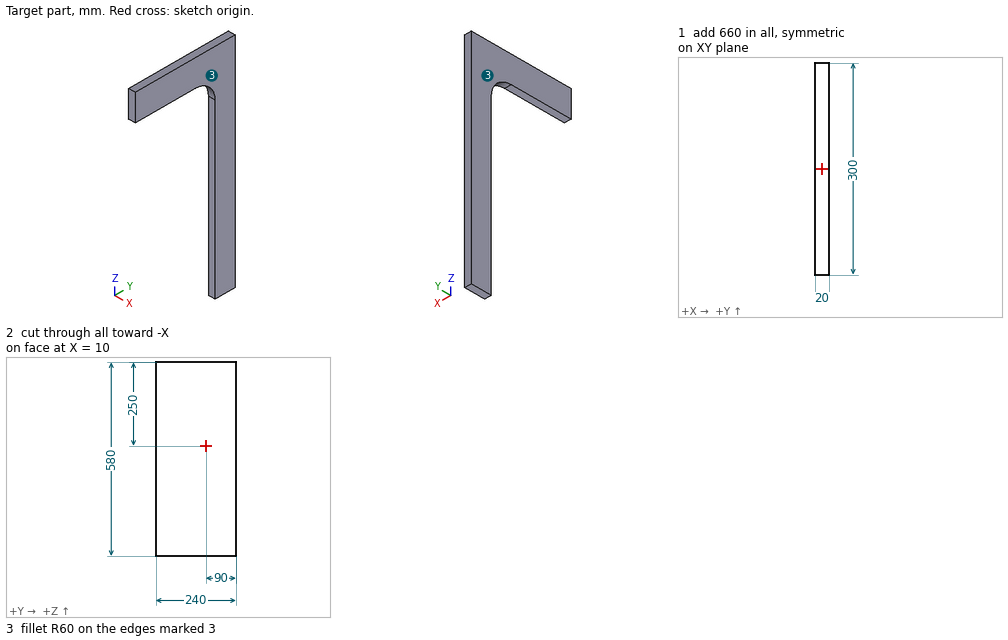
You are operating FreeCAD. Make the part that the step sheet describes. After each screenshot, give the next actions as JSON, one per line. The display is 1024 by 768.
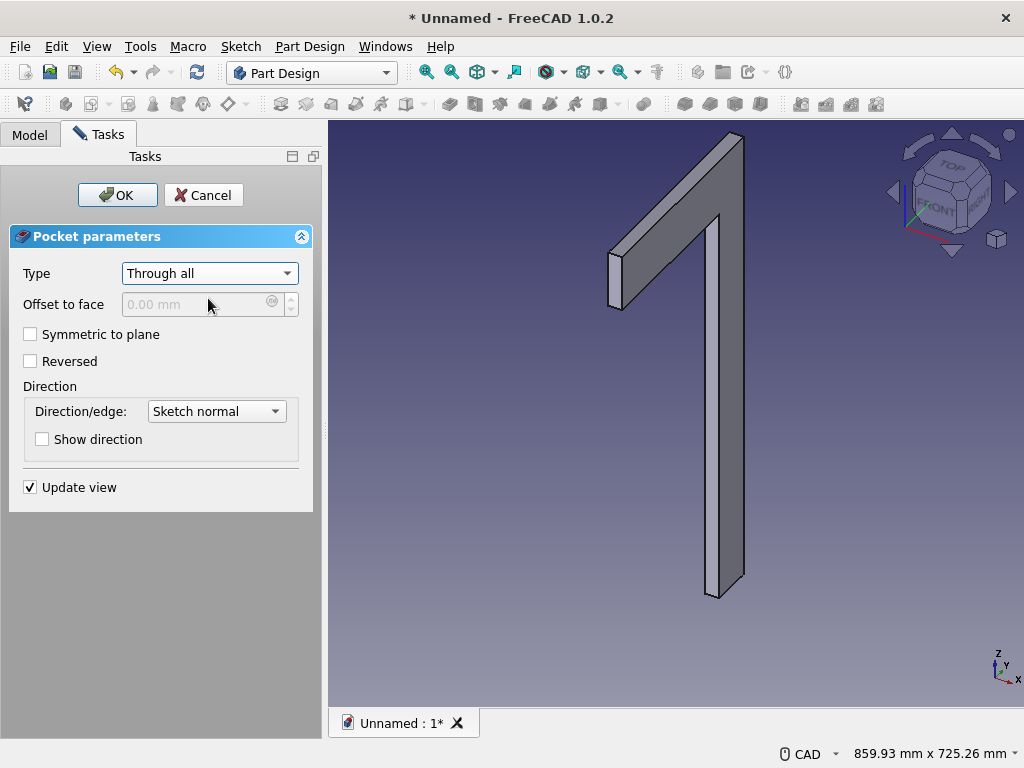
{"action": "left_click", "coordinate": [118, 195]}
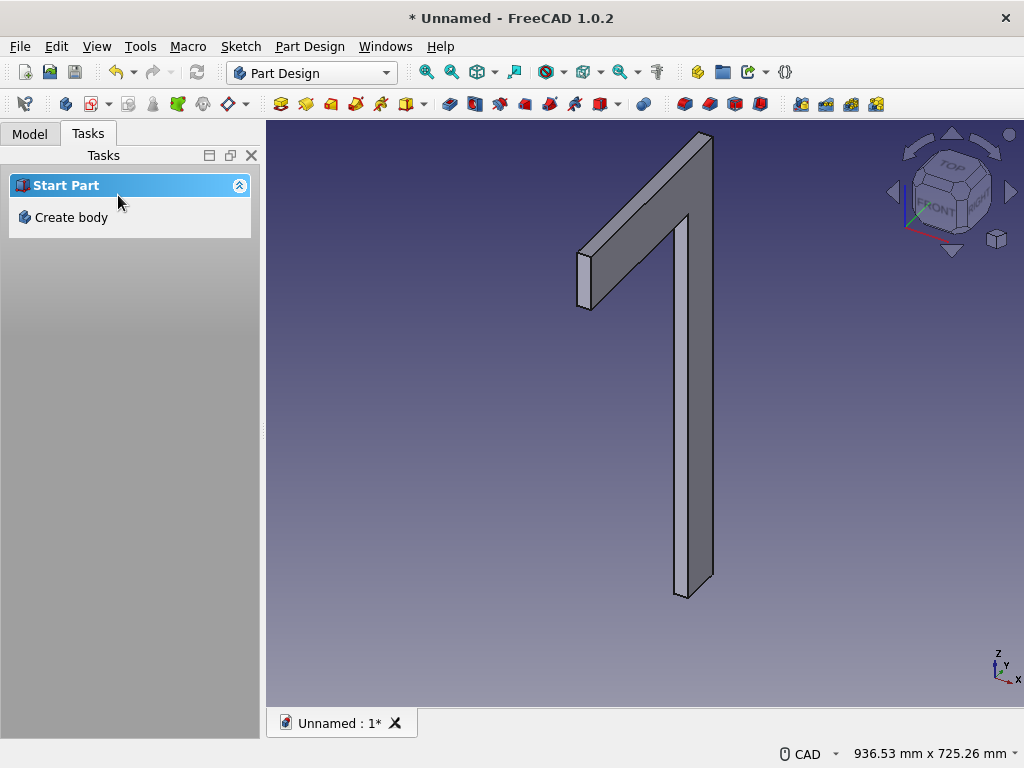
{"action": "scroll", "coordinate": [681, 211], "scroll_direction": "up", "scroll_amount": 5}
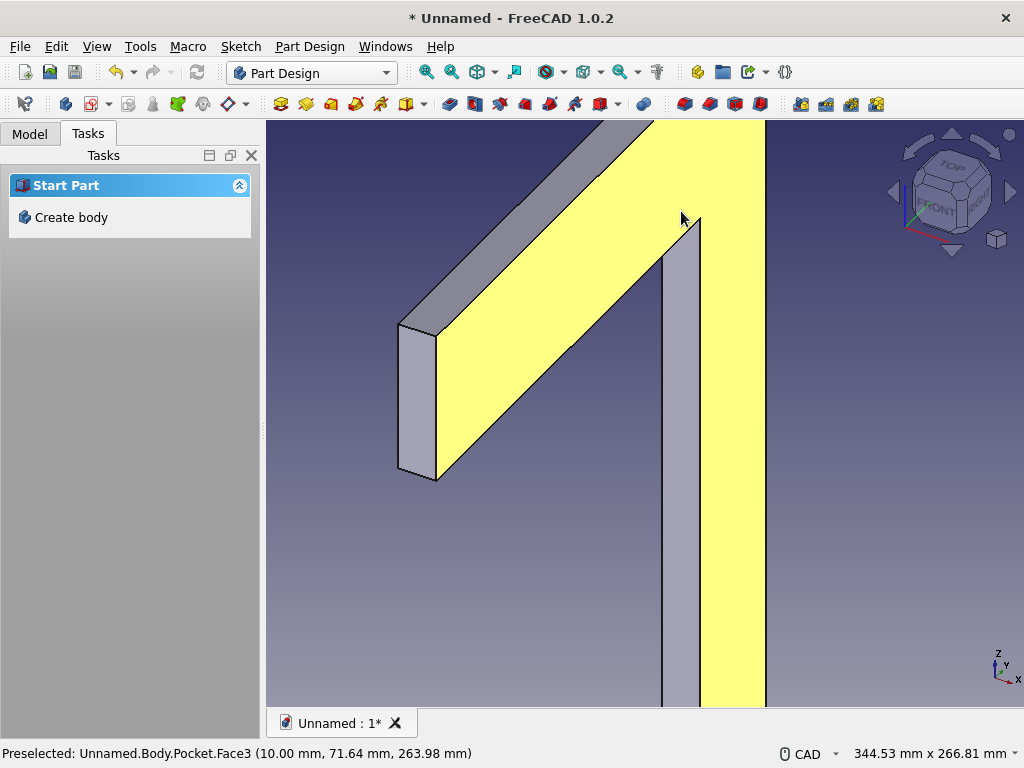
{"action": "left_click", "coordinate": [427, 72]}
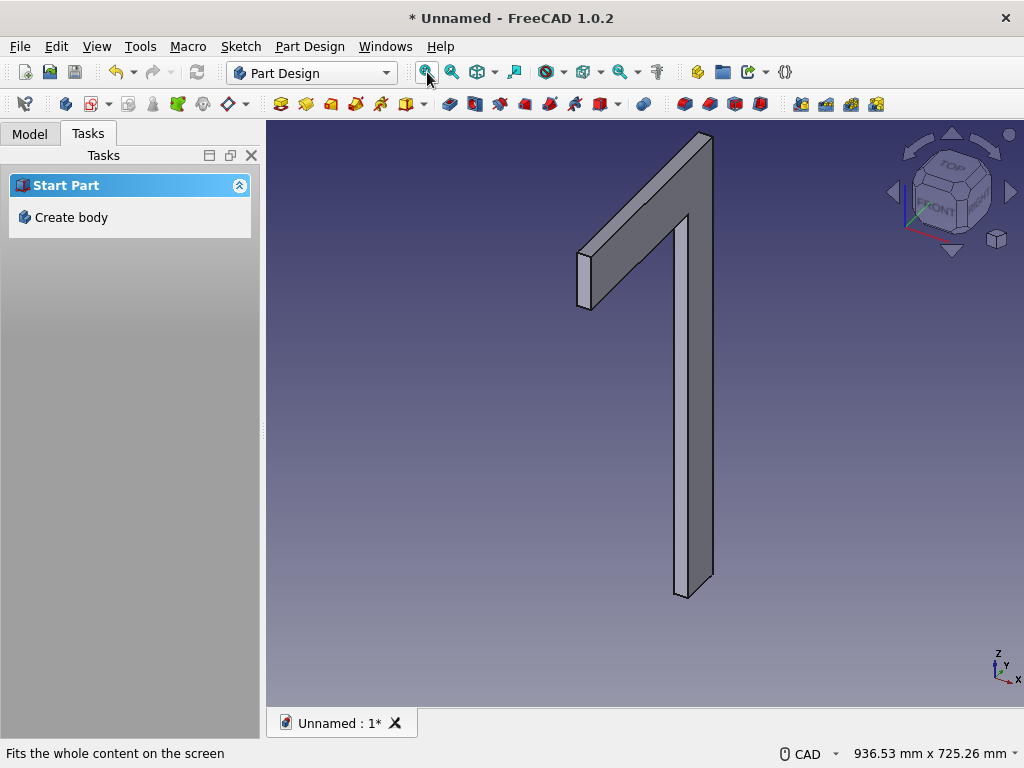
{"action": "key", "text": "0"}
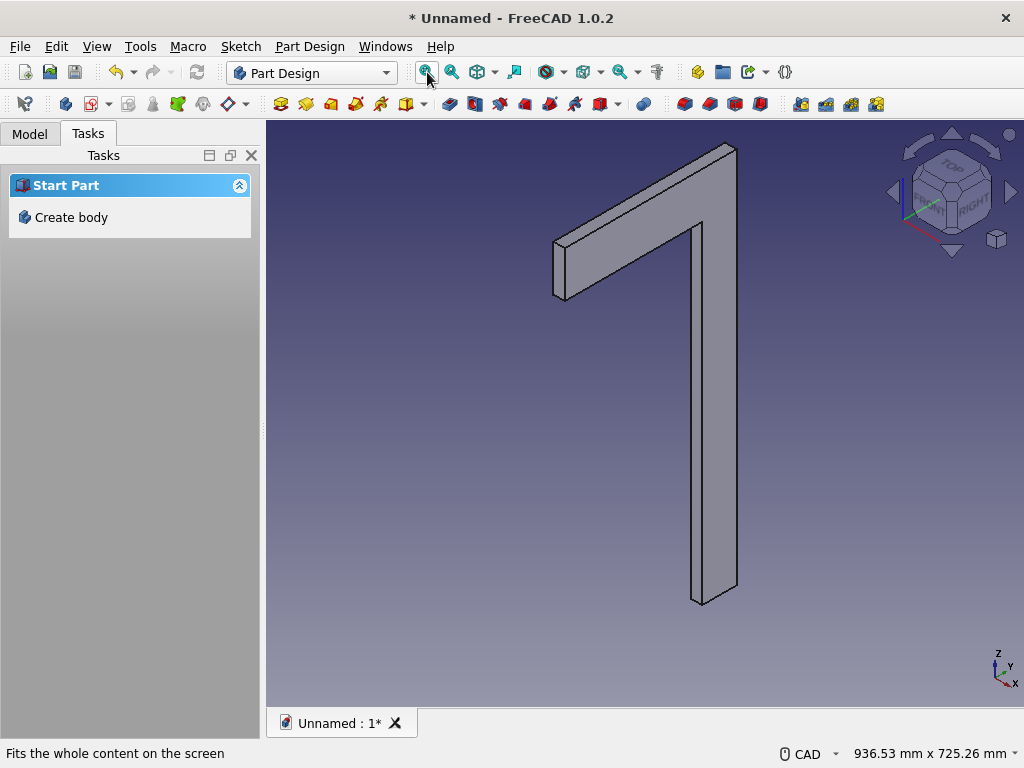
{"action": "scroll", "coordinate": [697, 218], "scroll_direction": "up", "scroll_amount": 5}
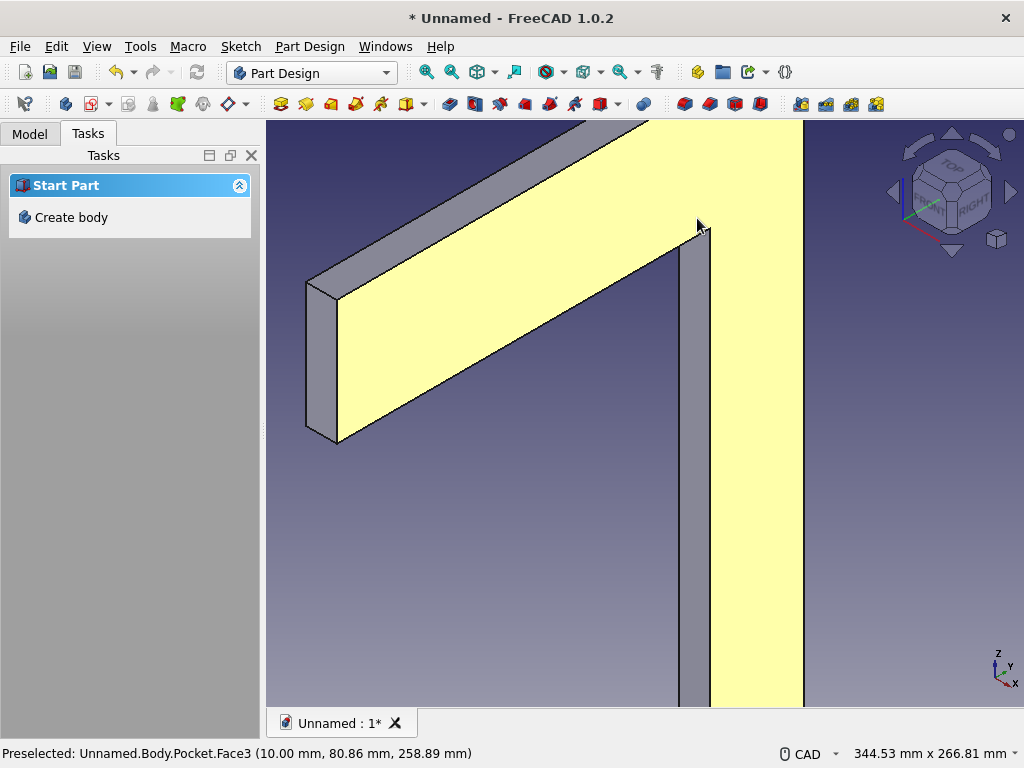
{"action": "left_click", "coordinate": [427, 72]}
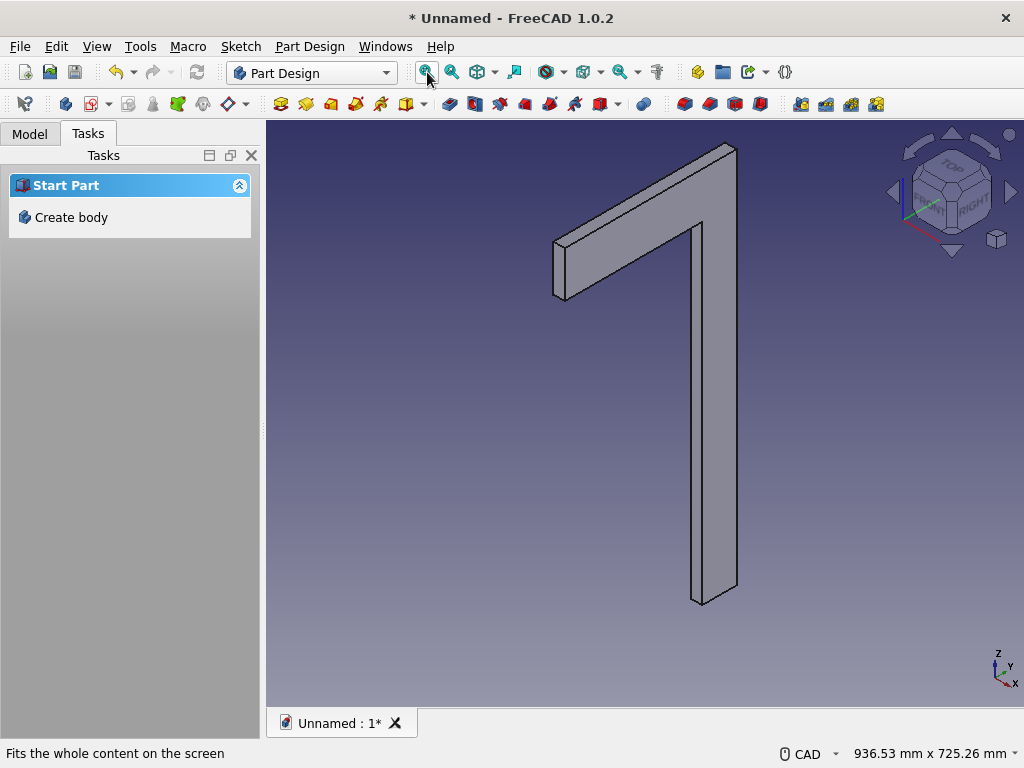
{"action": "key", "text": "2"}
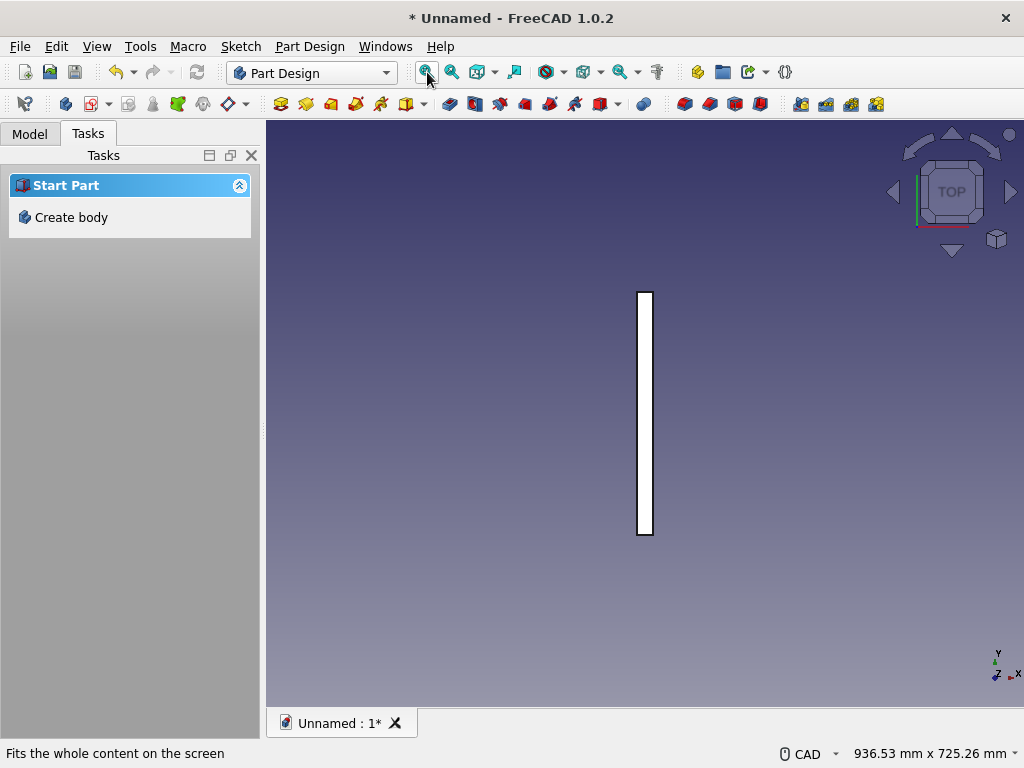
{"action": "left_click", "coordinate": [427, 72]}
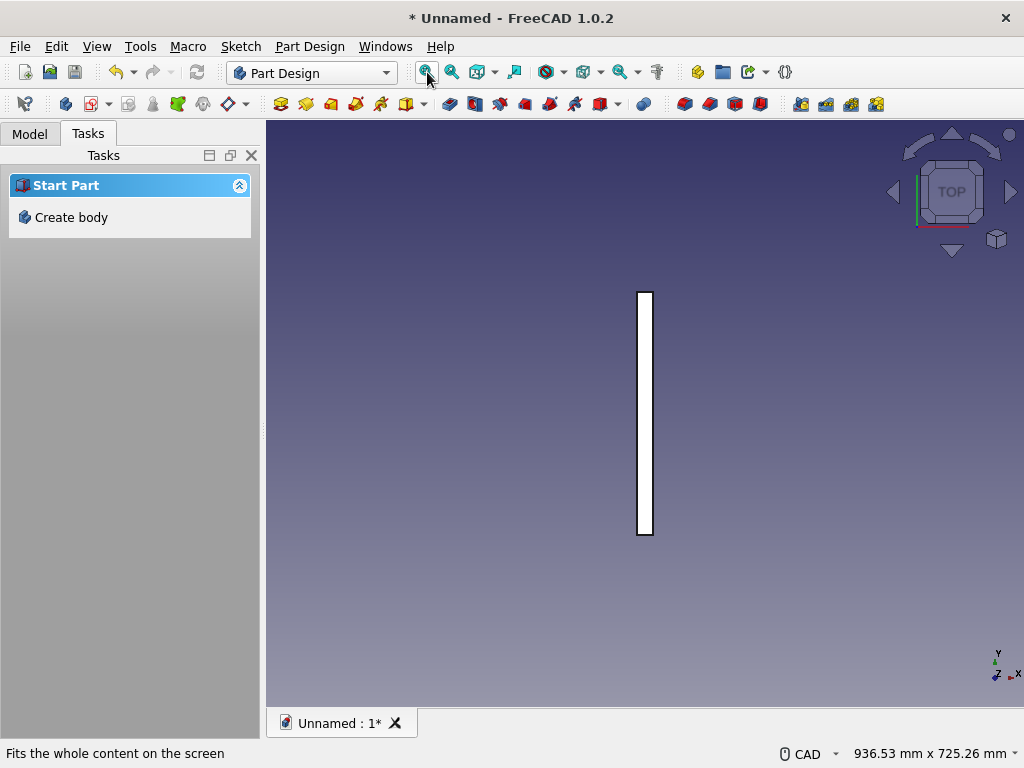
{"action": "scroll", "coordinate": [645, 340], "scroll_direction": "up", "scroll_amount": 5}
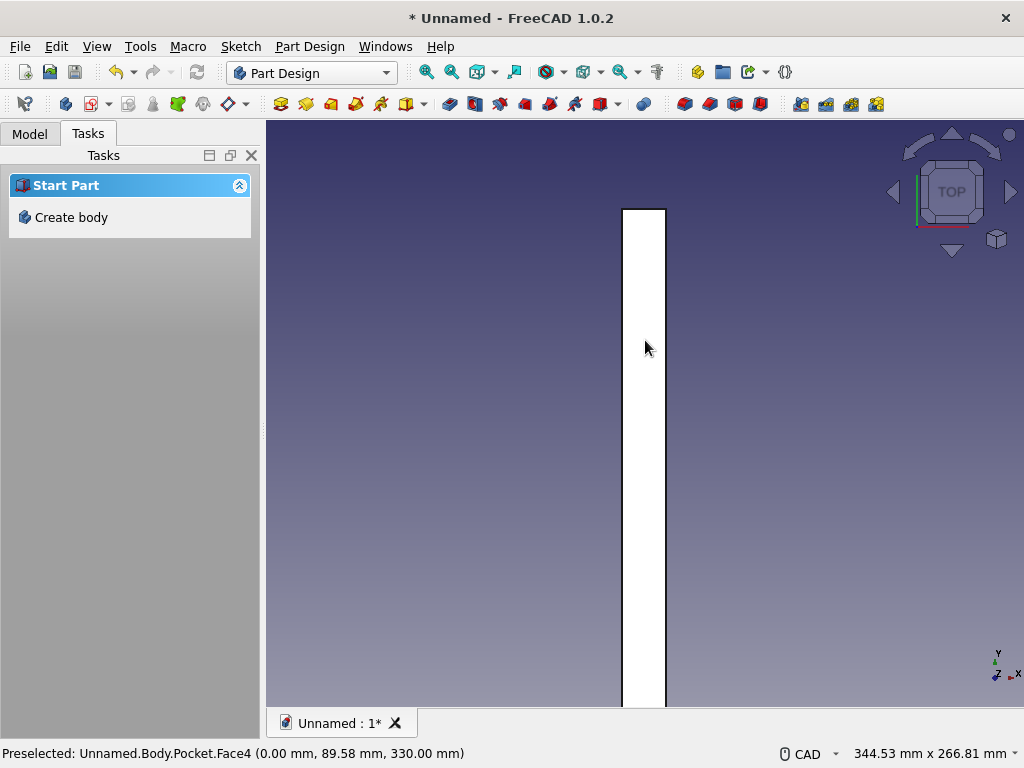
{"action": "key", "text": "v f"}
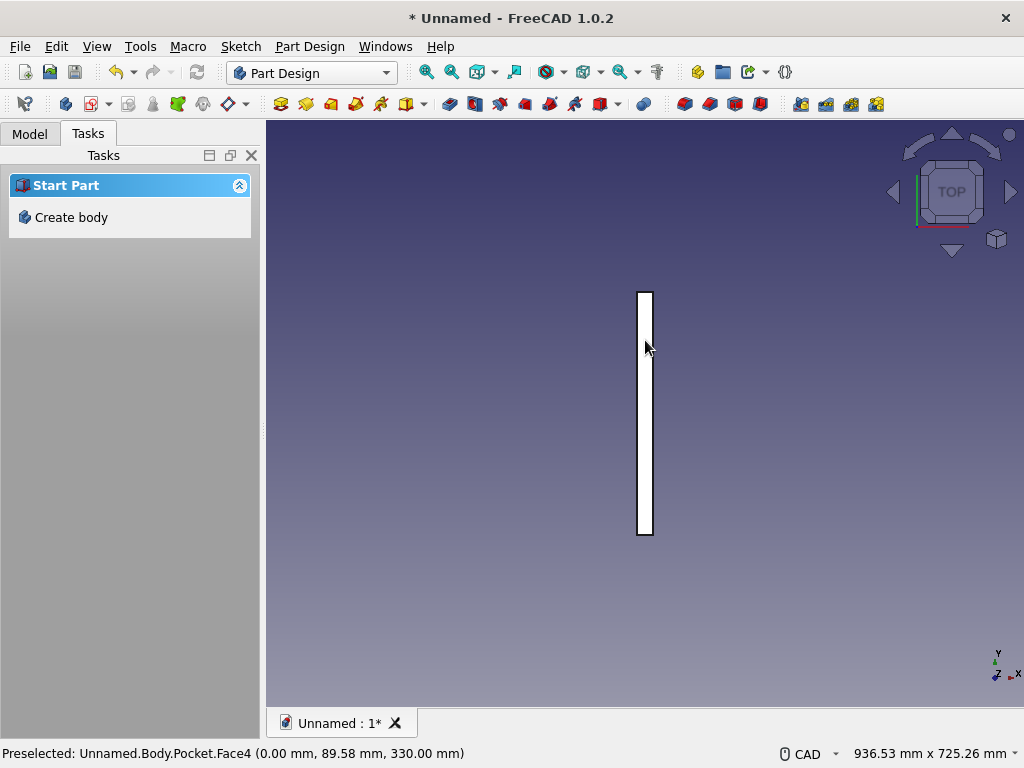
{"action": "key", "text": "1"}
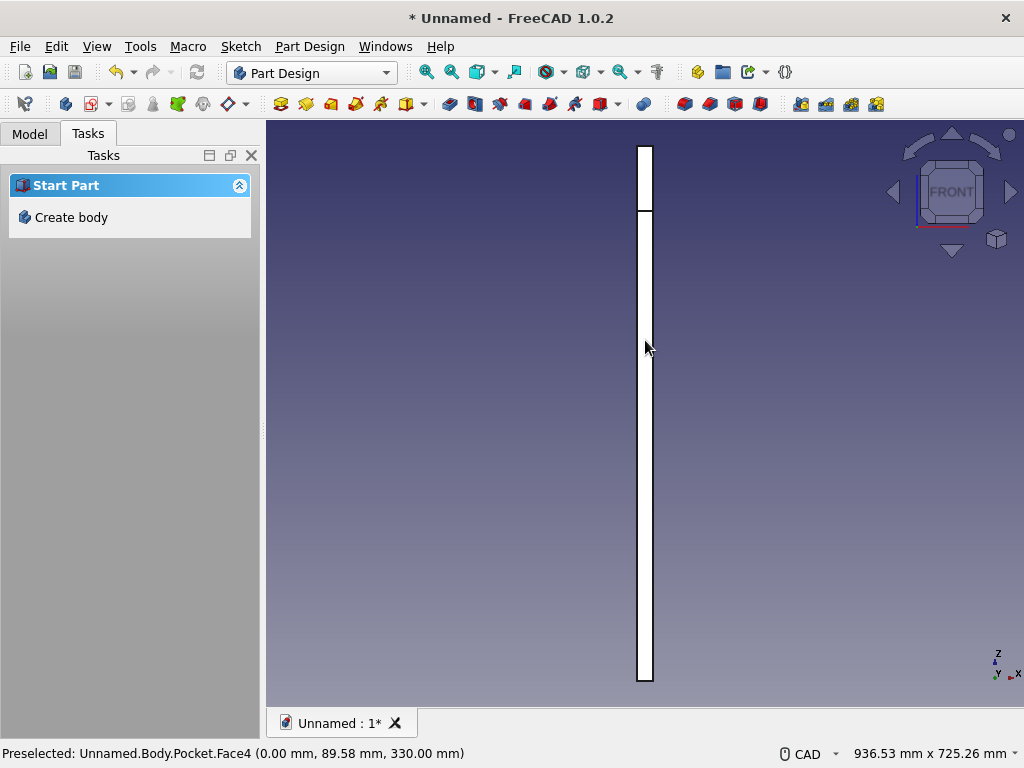
{"action": "scroll", "coordinate": [645, 210], "scroll_direction": "up", "scroll_amount": 5}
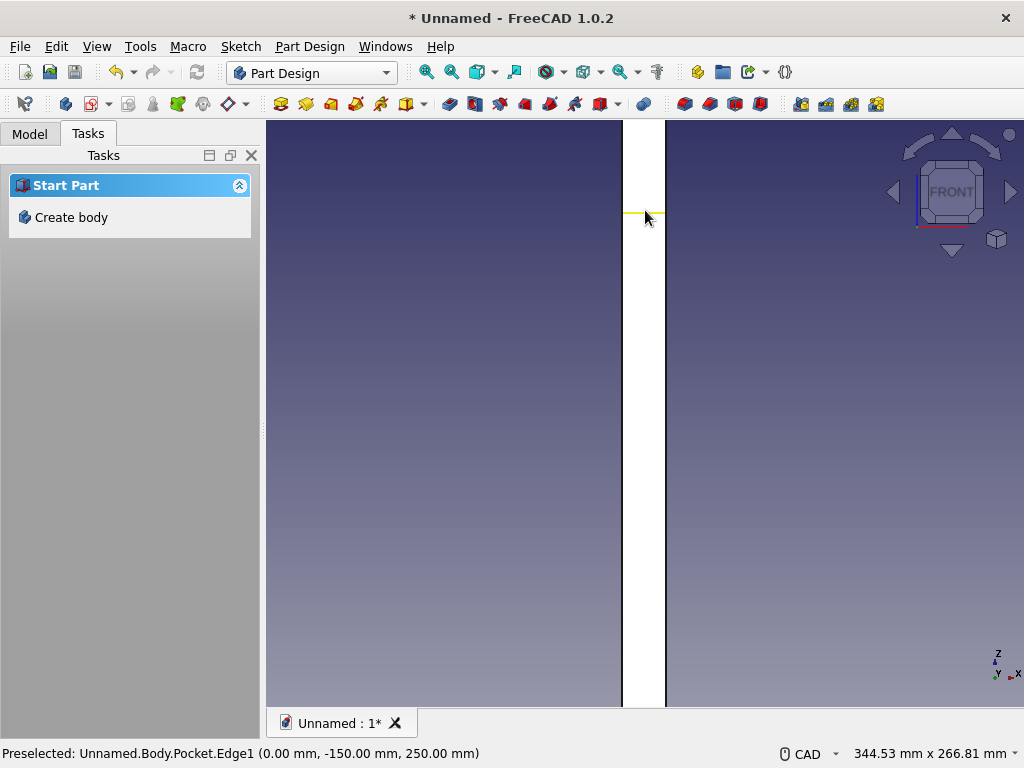
{"action": "left_click", "coordinate": [427, 72]}